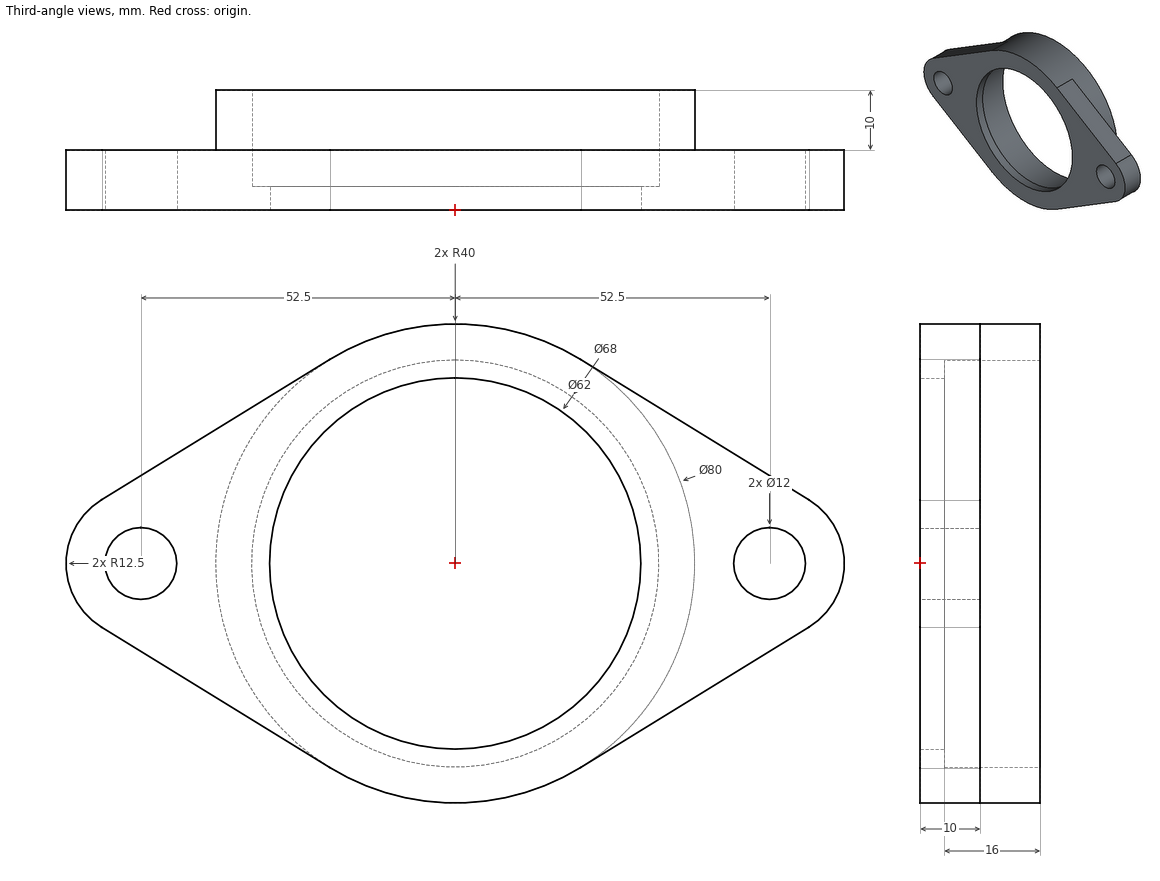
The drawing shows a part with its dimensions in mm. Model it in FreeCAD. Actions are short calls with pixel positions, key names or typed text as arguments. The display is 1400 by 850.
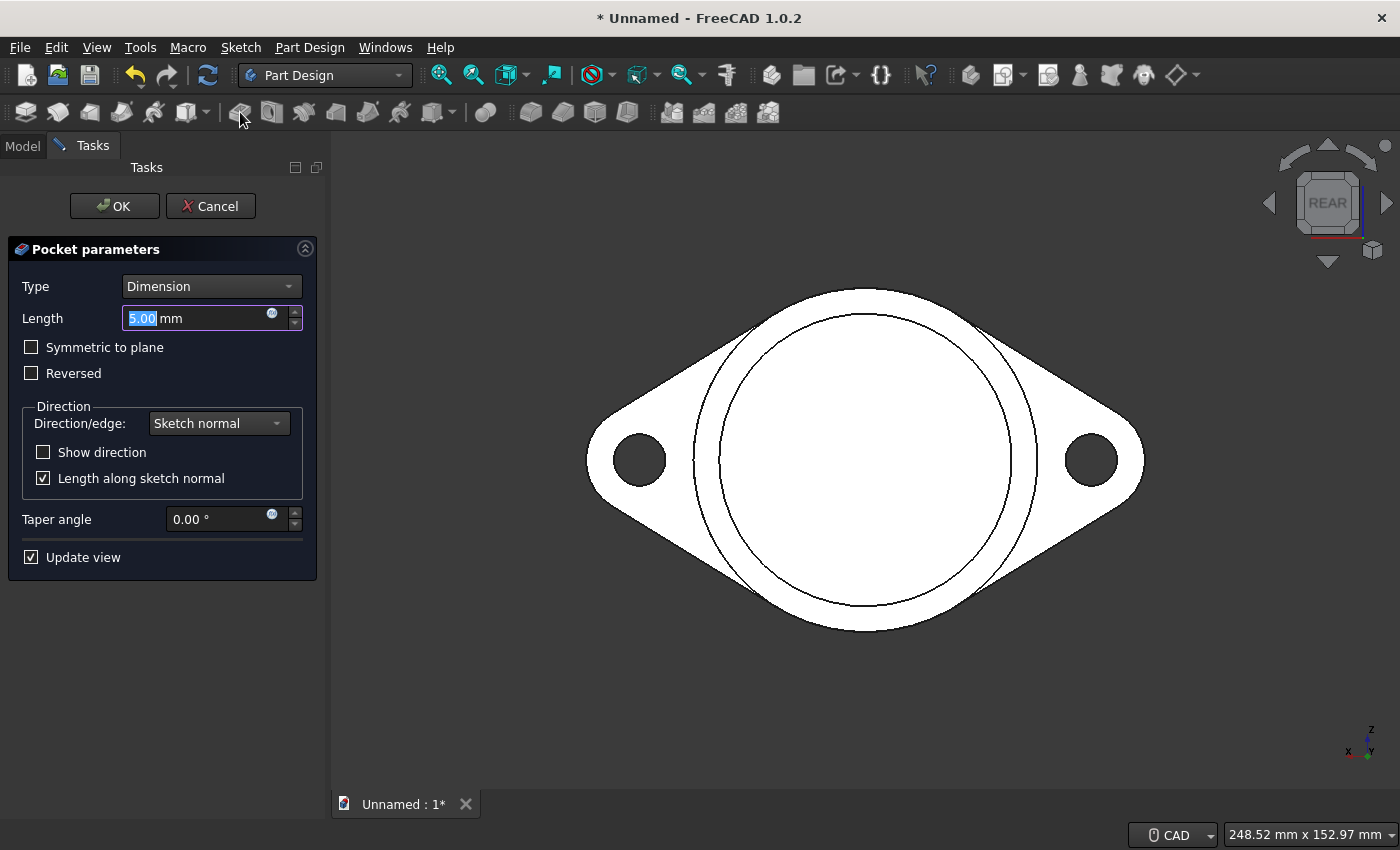
text(16)
key(Tab)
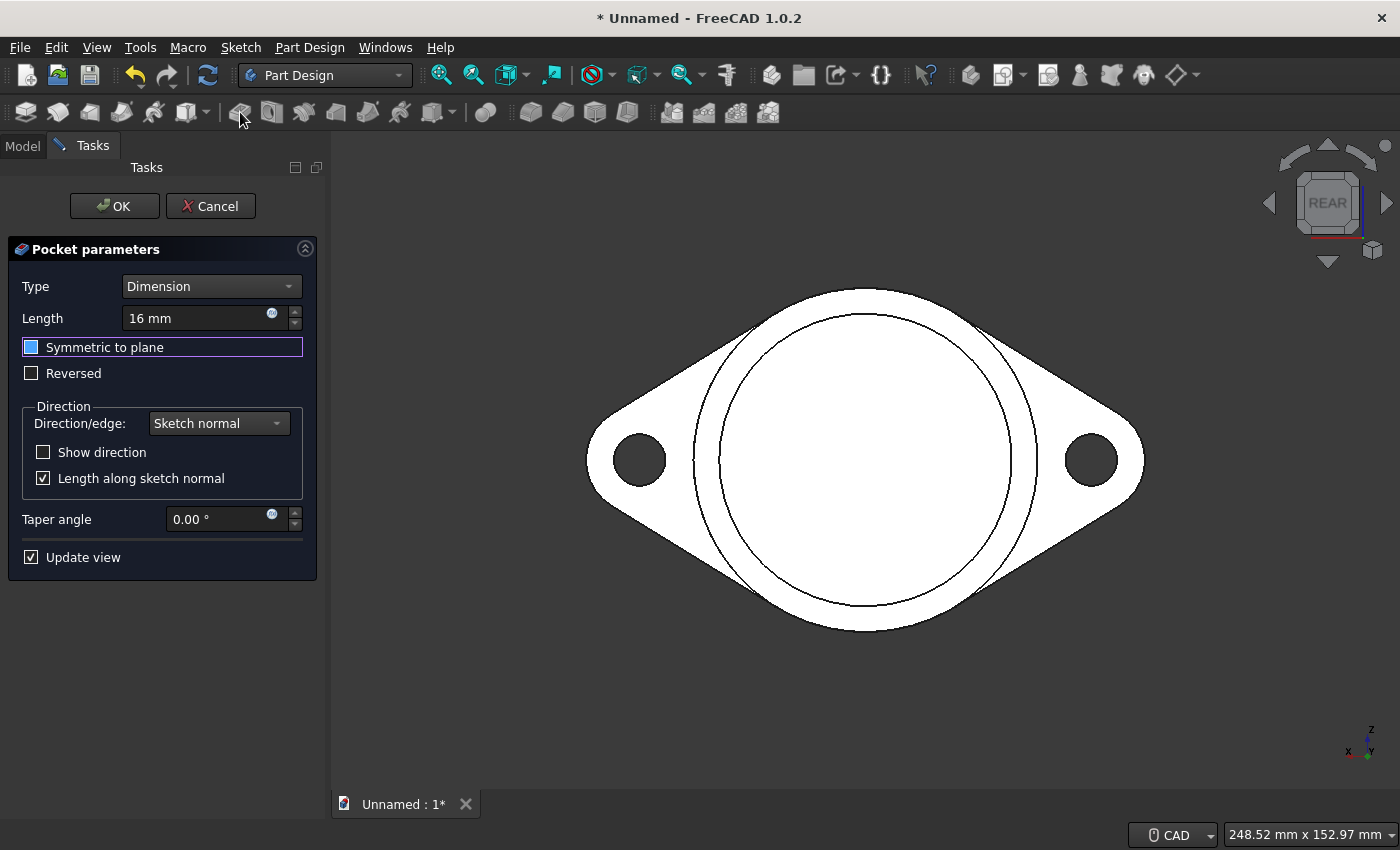
click(115, 206)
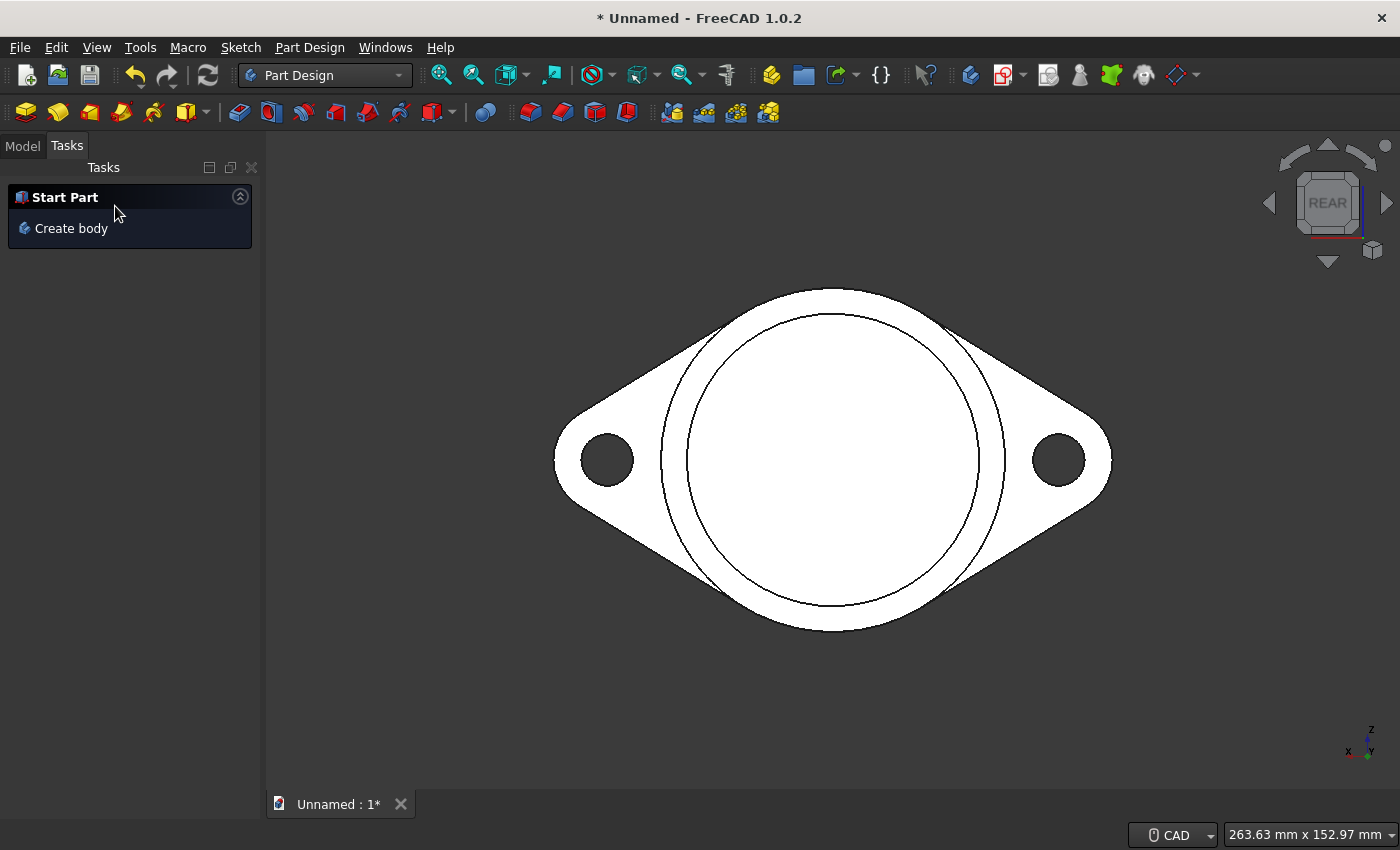
click(833, 459)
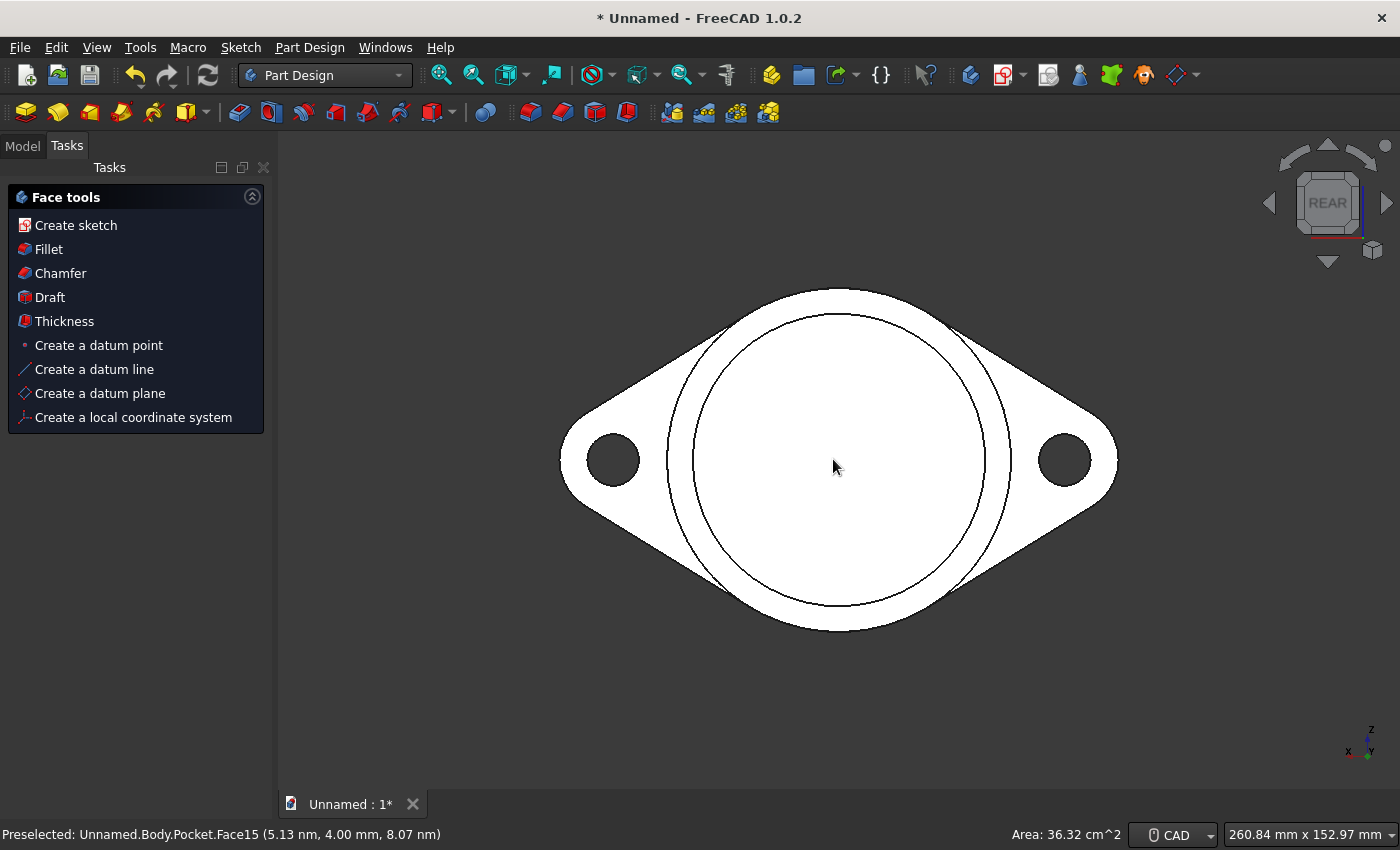
click(1004, 76)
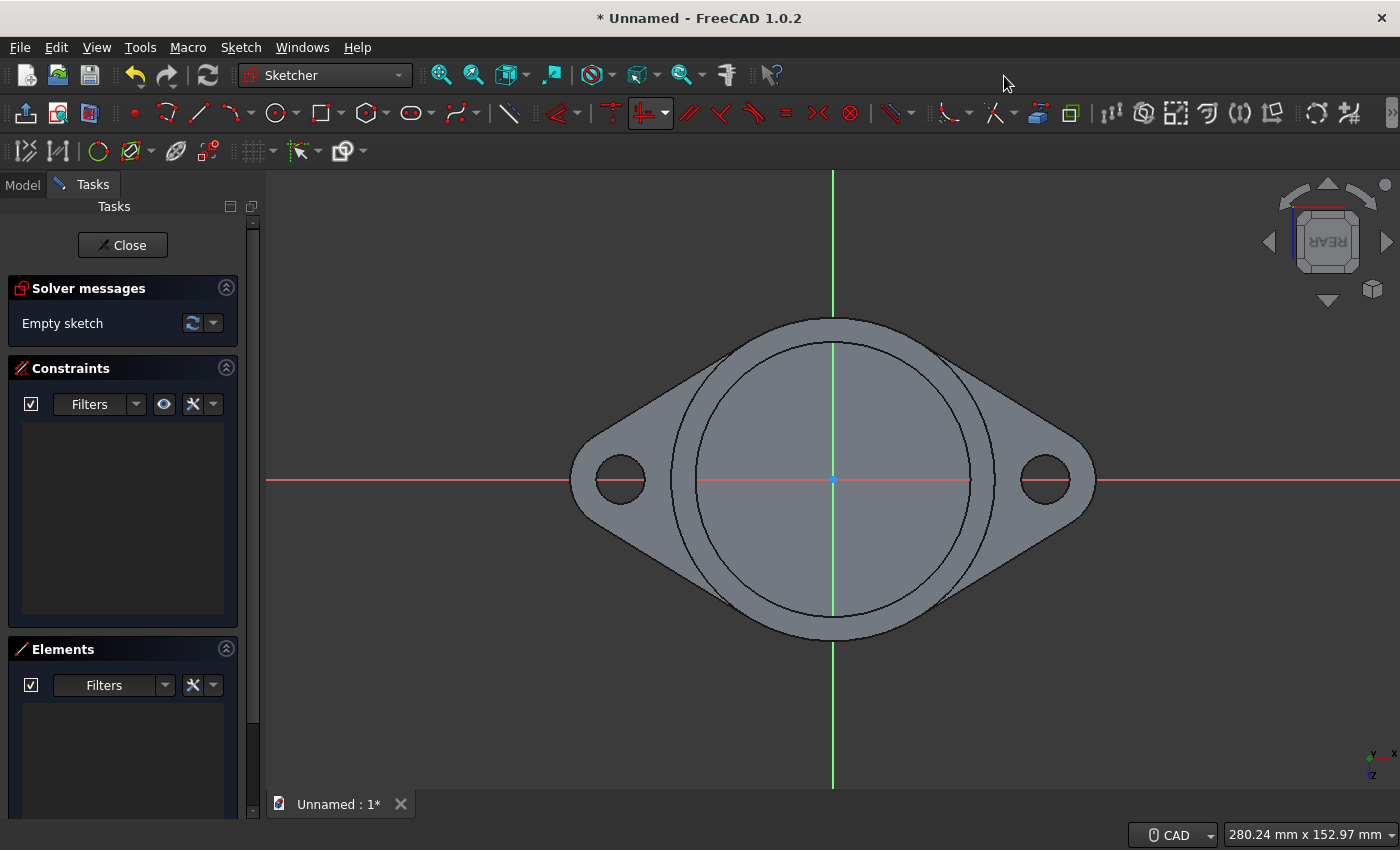
scroll(972, 479, up, 2)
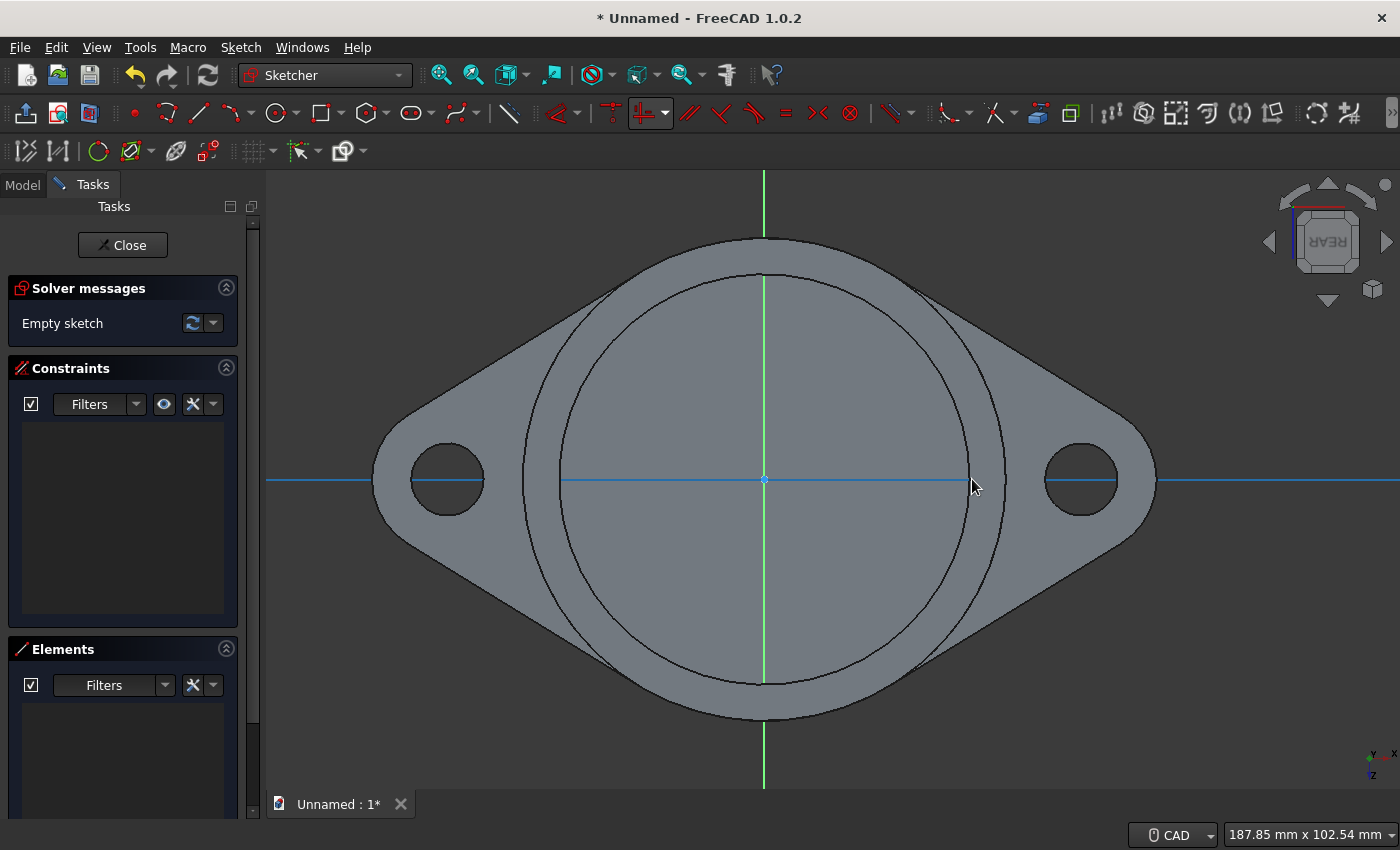
click(276, 114)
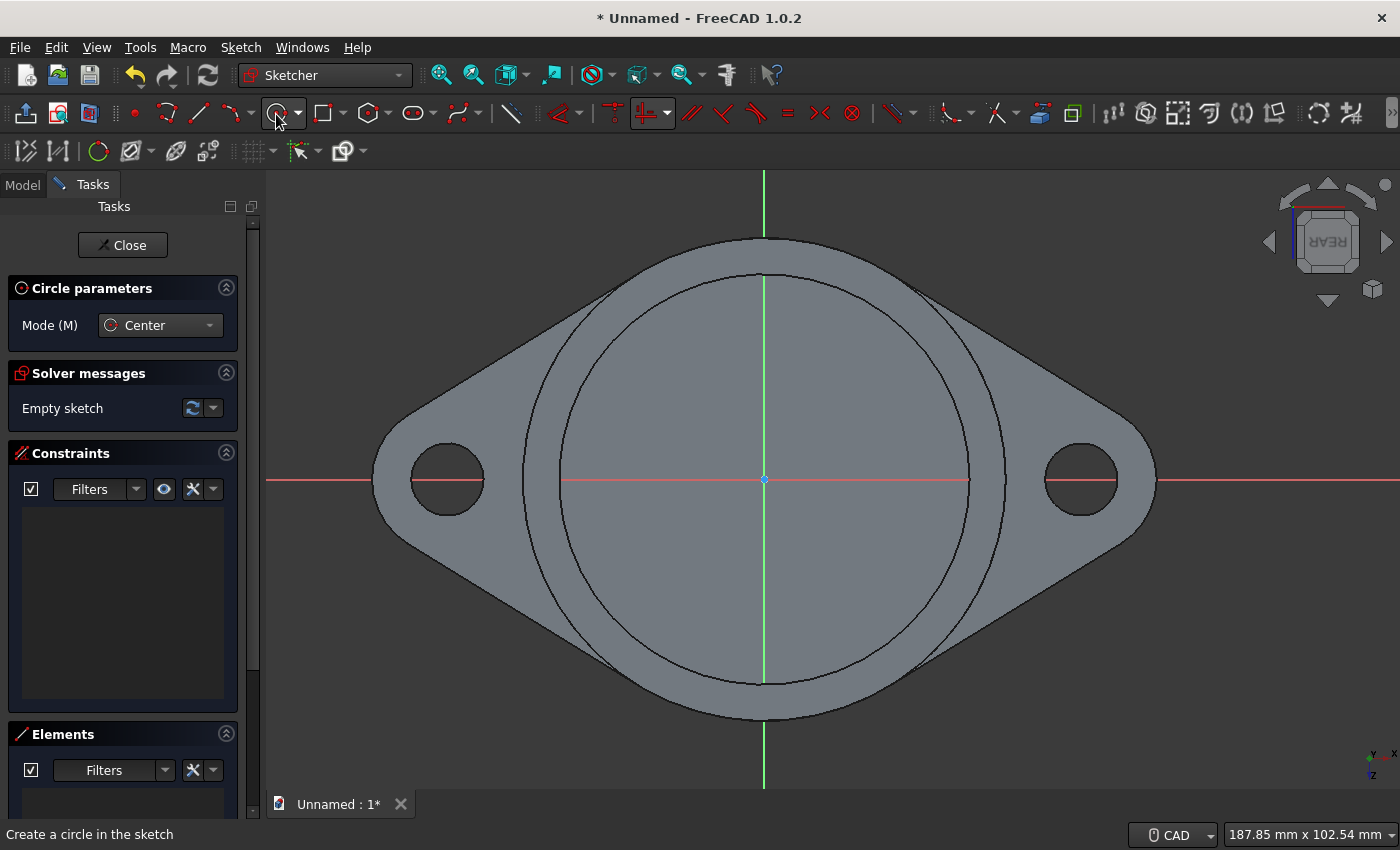
click(764, 479)
move(897, 347)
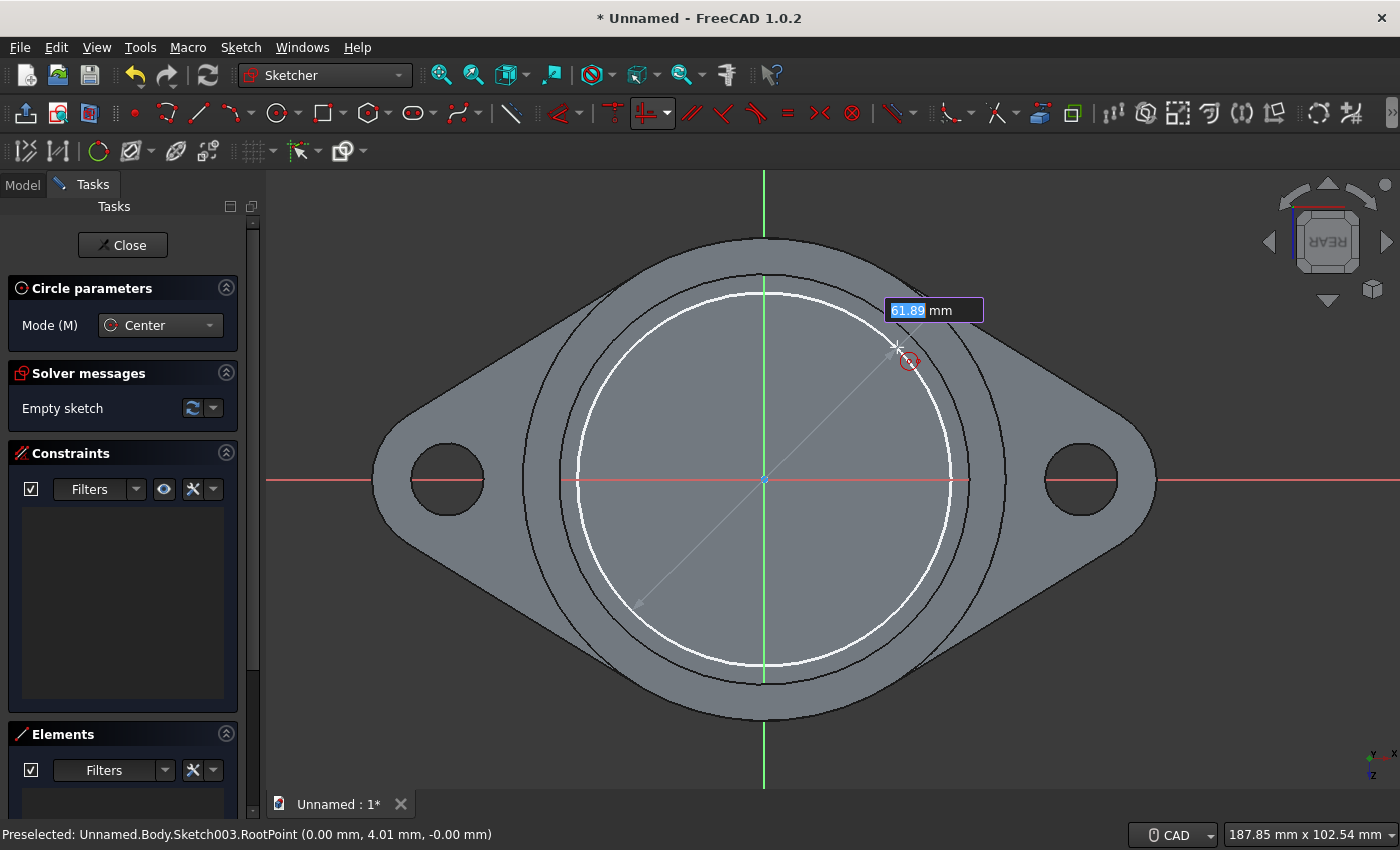
text(62)
key(Return)
key(Escape)